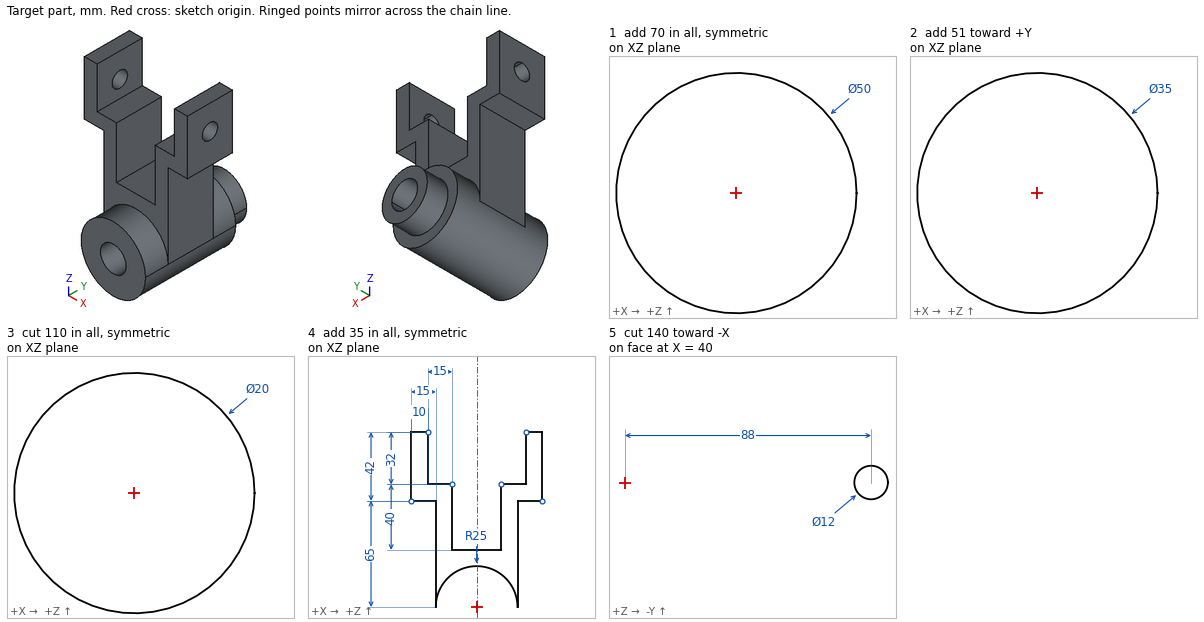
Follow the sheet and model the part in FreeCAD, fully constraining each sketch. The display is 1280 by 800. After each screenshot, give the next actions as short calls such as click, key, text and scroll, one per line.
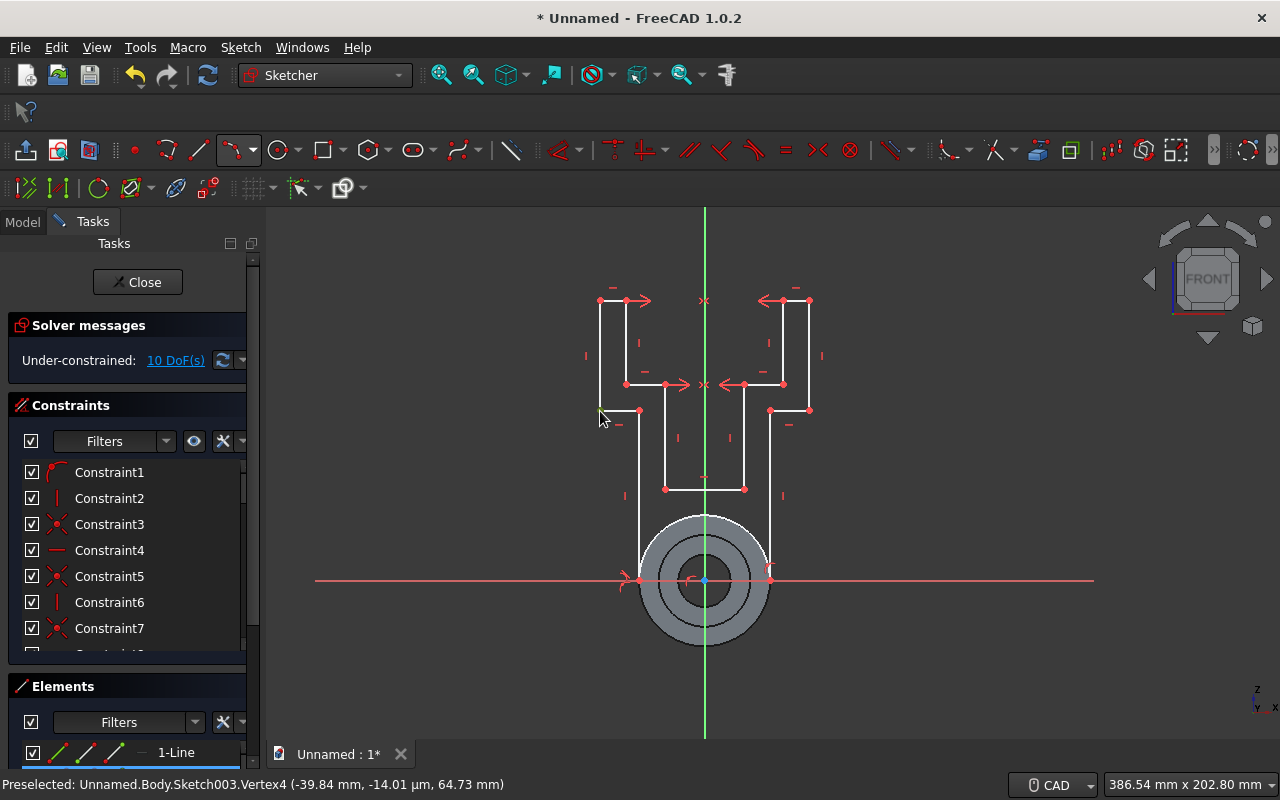
click(809, 411)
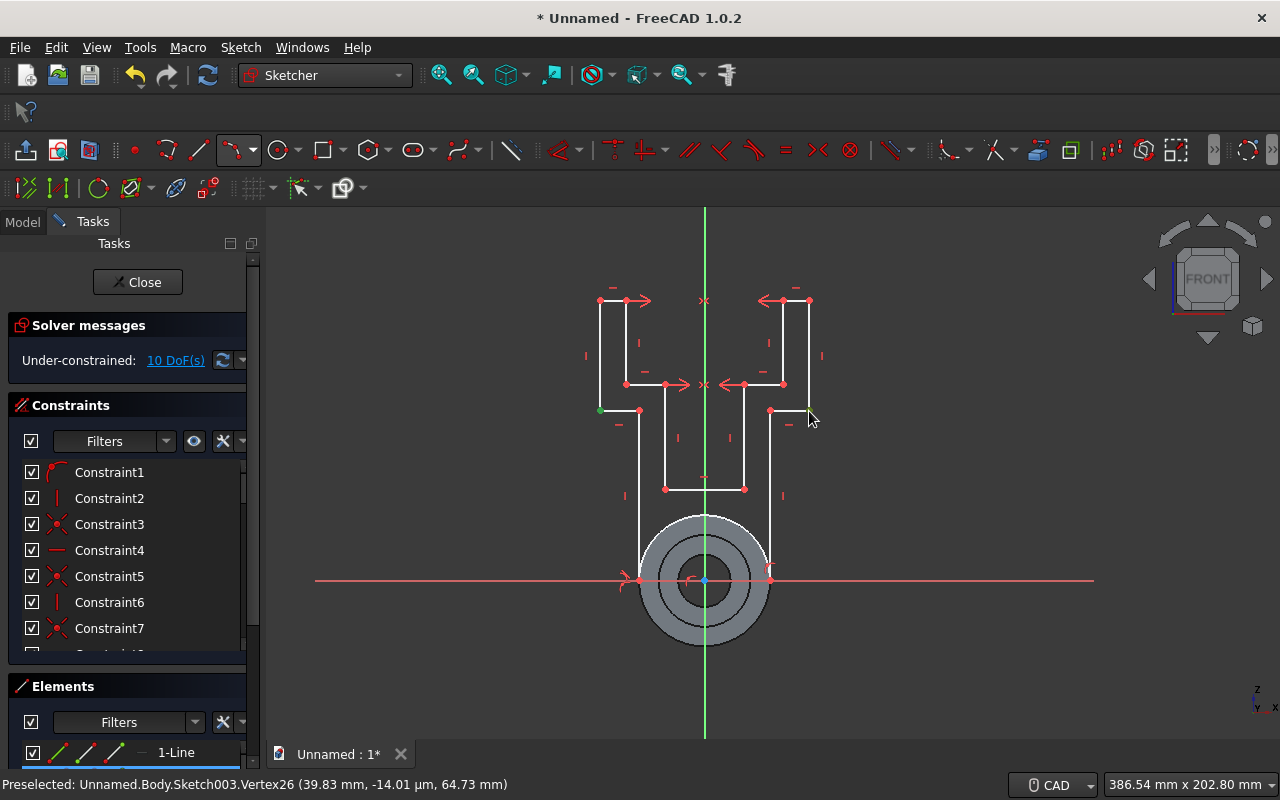
click(705, 677)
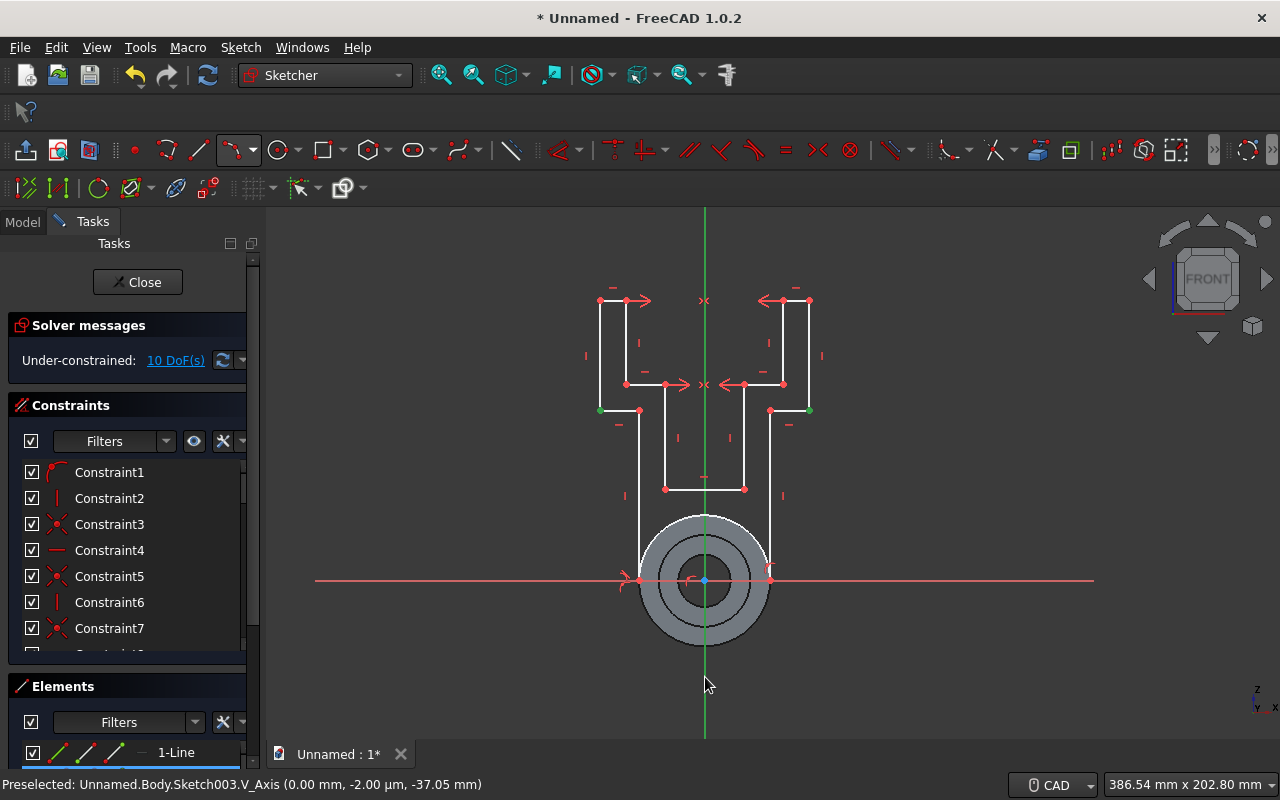
click(818, 150)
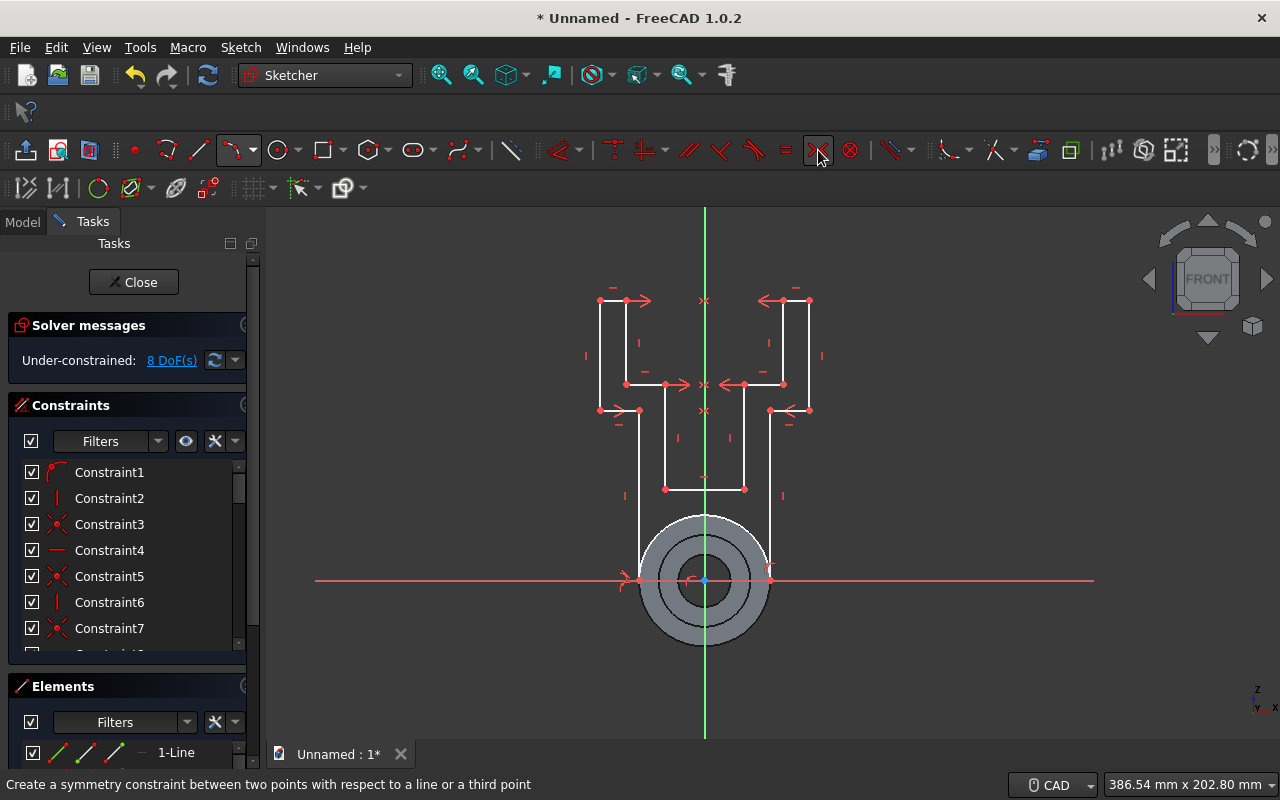
click(558, 150)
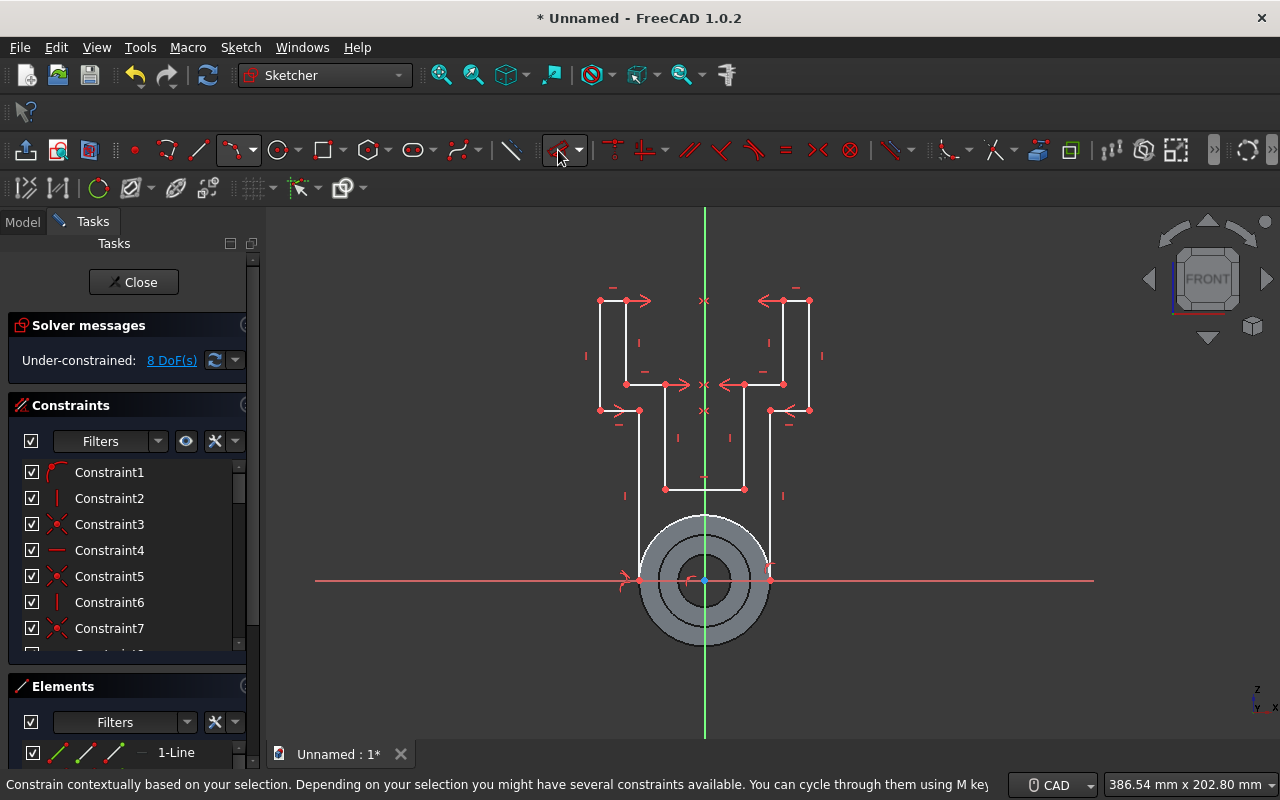
click(743, 528)
click(793, 539)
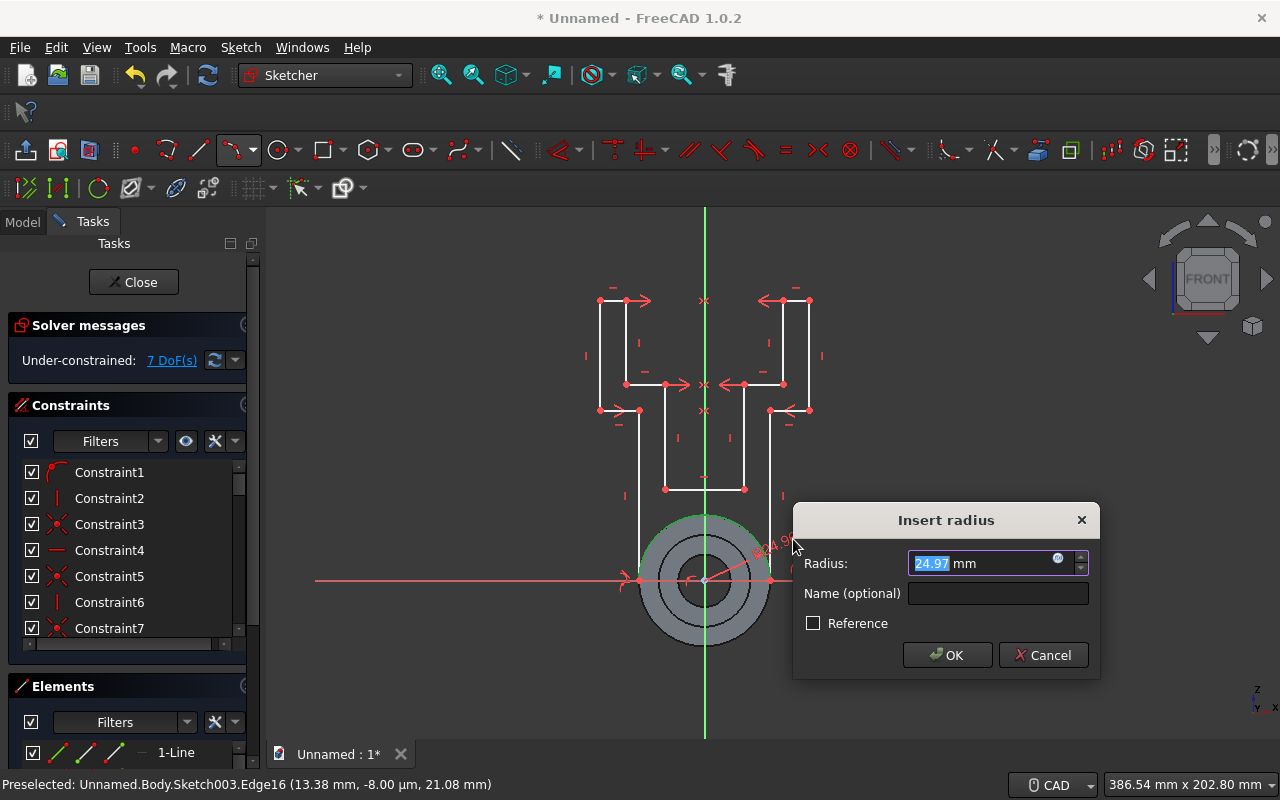
text(25)
key(Return)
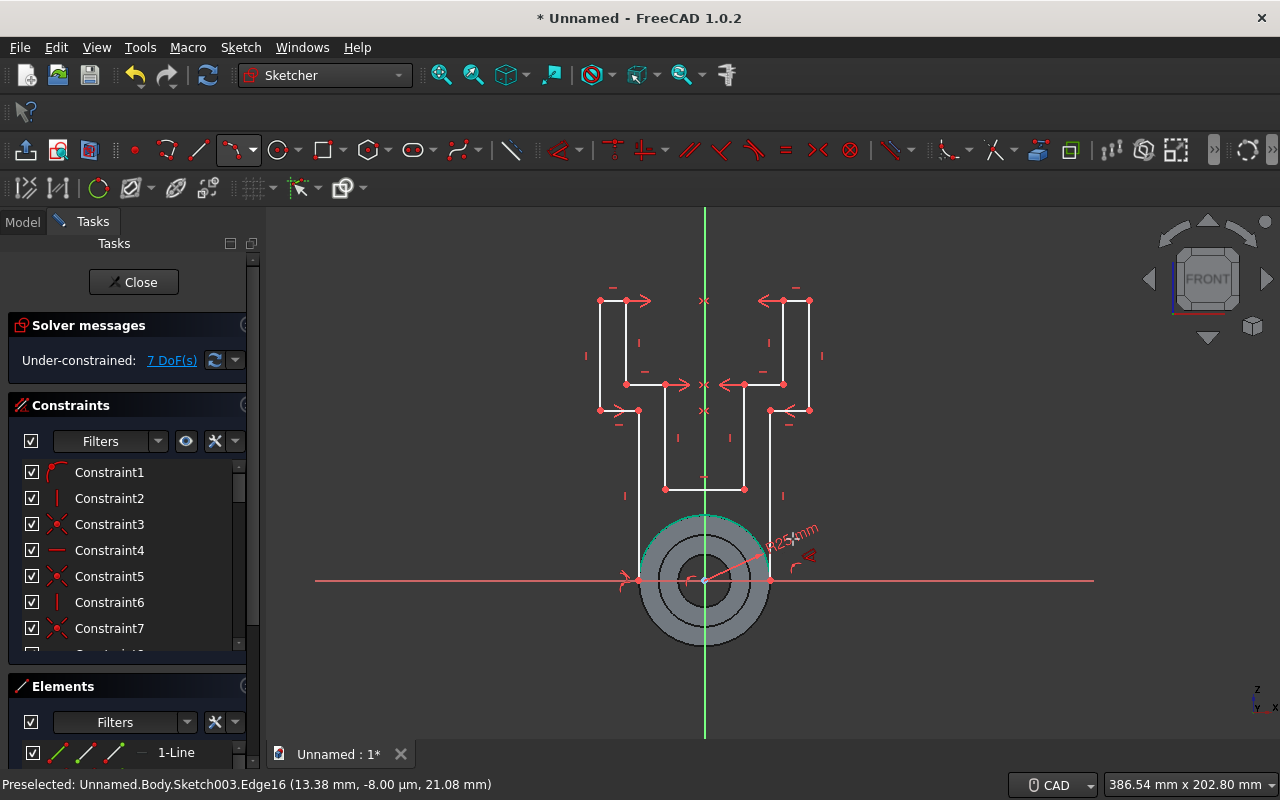
click(639, 530)
click(605, 496)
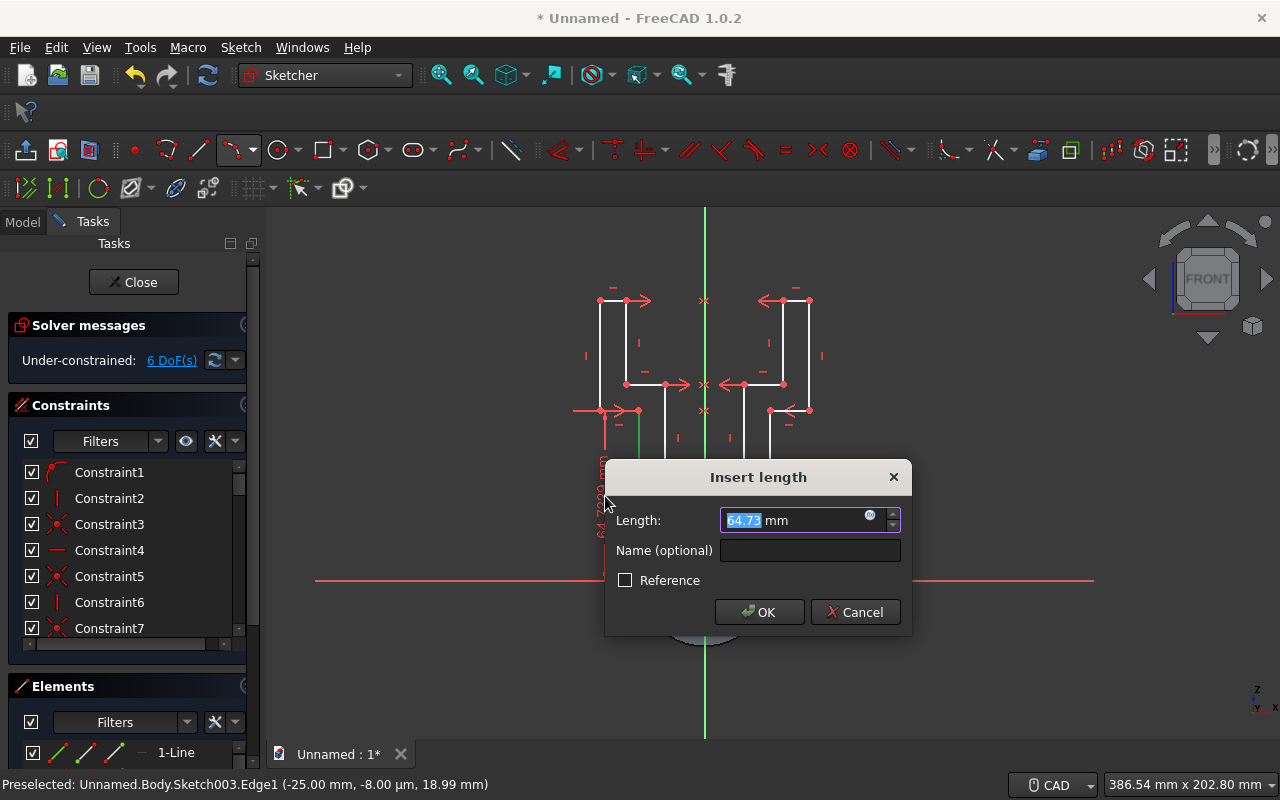
text(65)
key(Return)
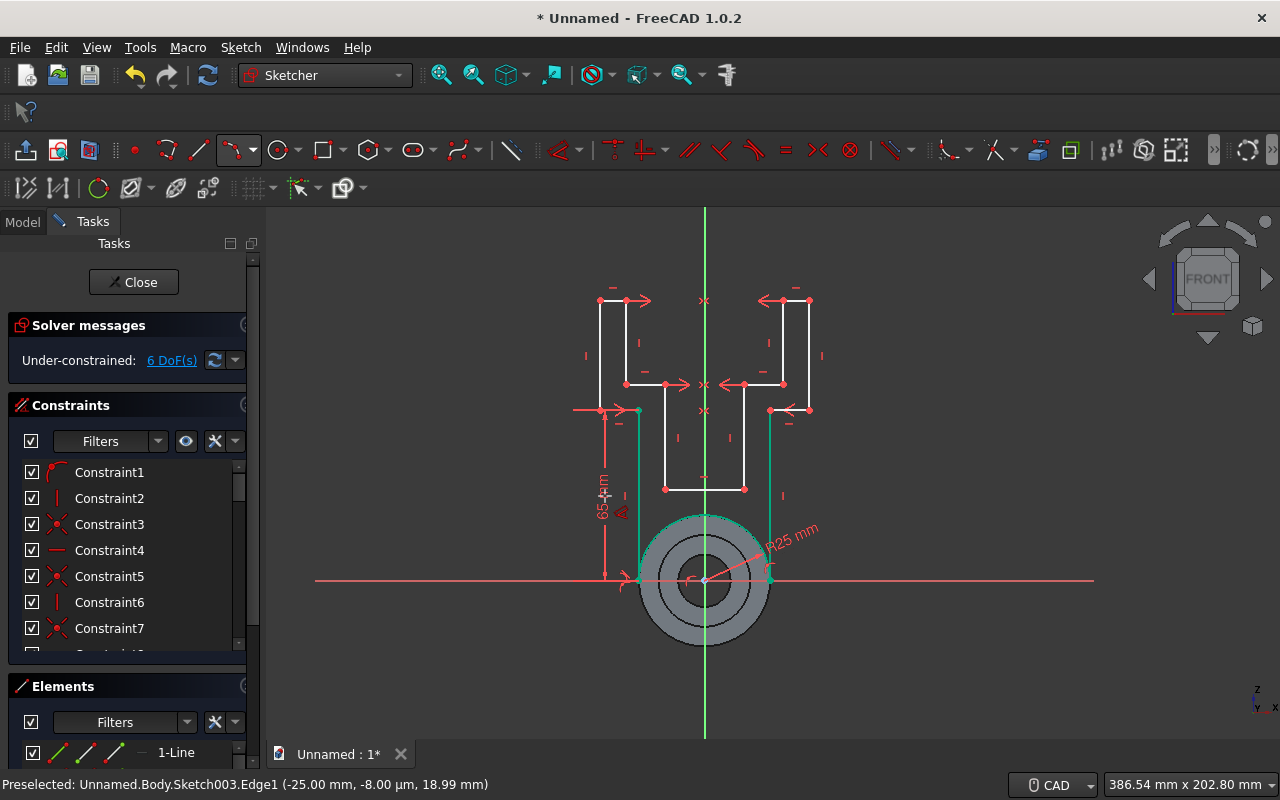
click(627, 410)
click(619, 444)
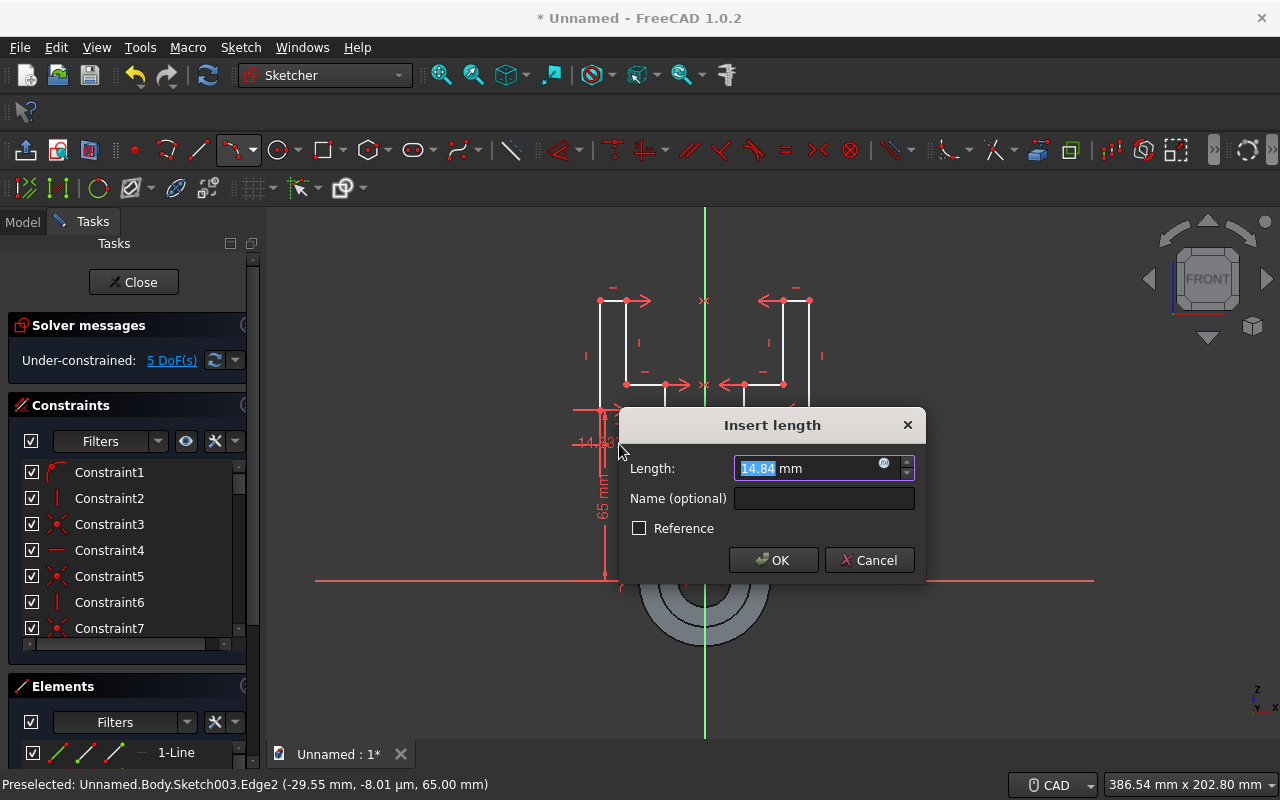
text(15)
key(Return)